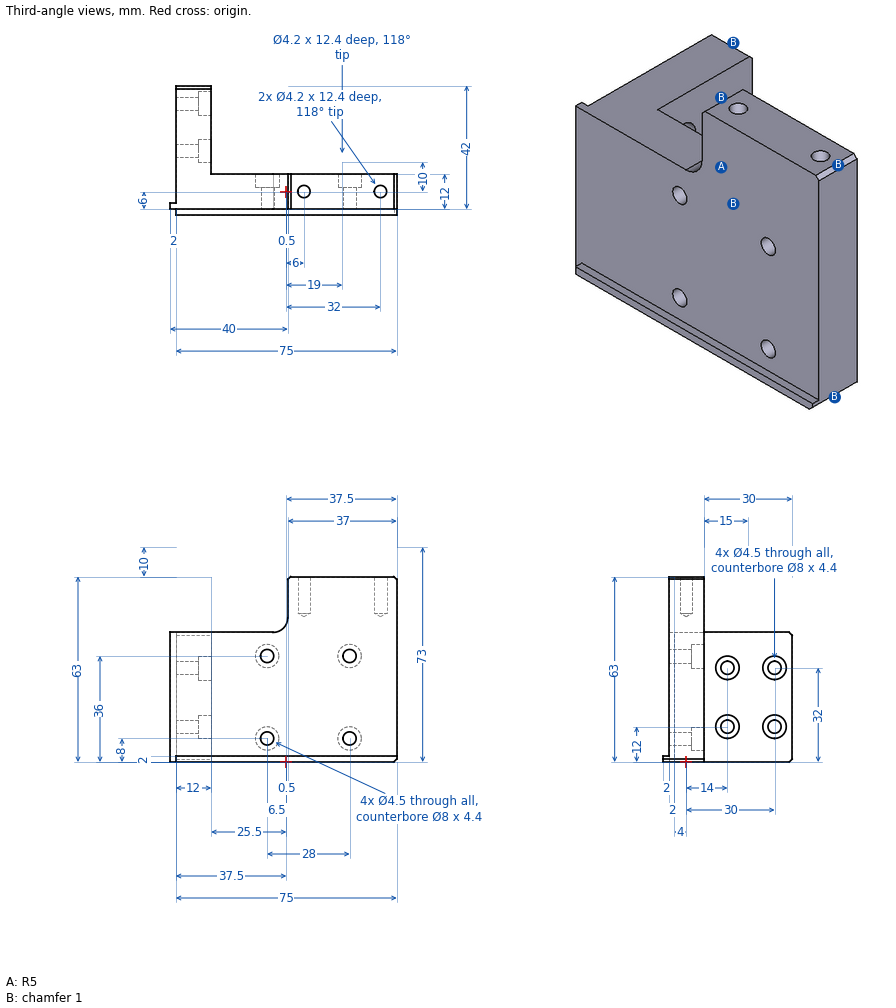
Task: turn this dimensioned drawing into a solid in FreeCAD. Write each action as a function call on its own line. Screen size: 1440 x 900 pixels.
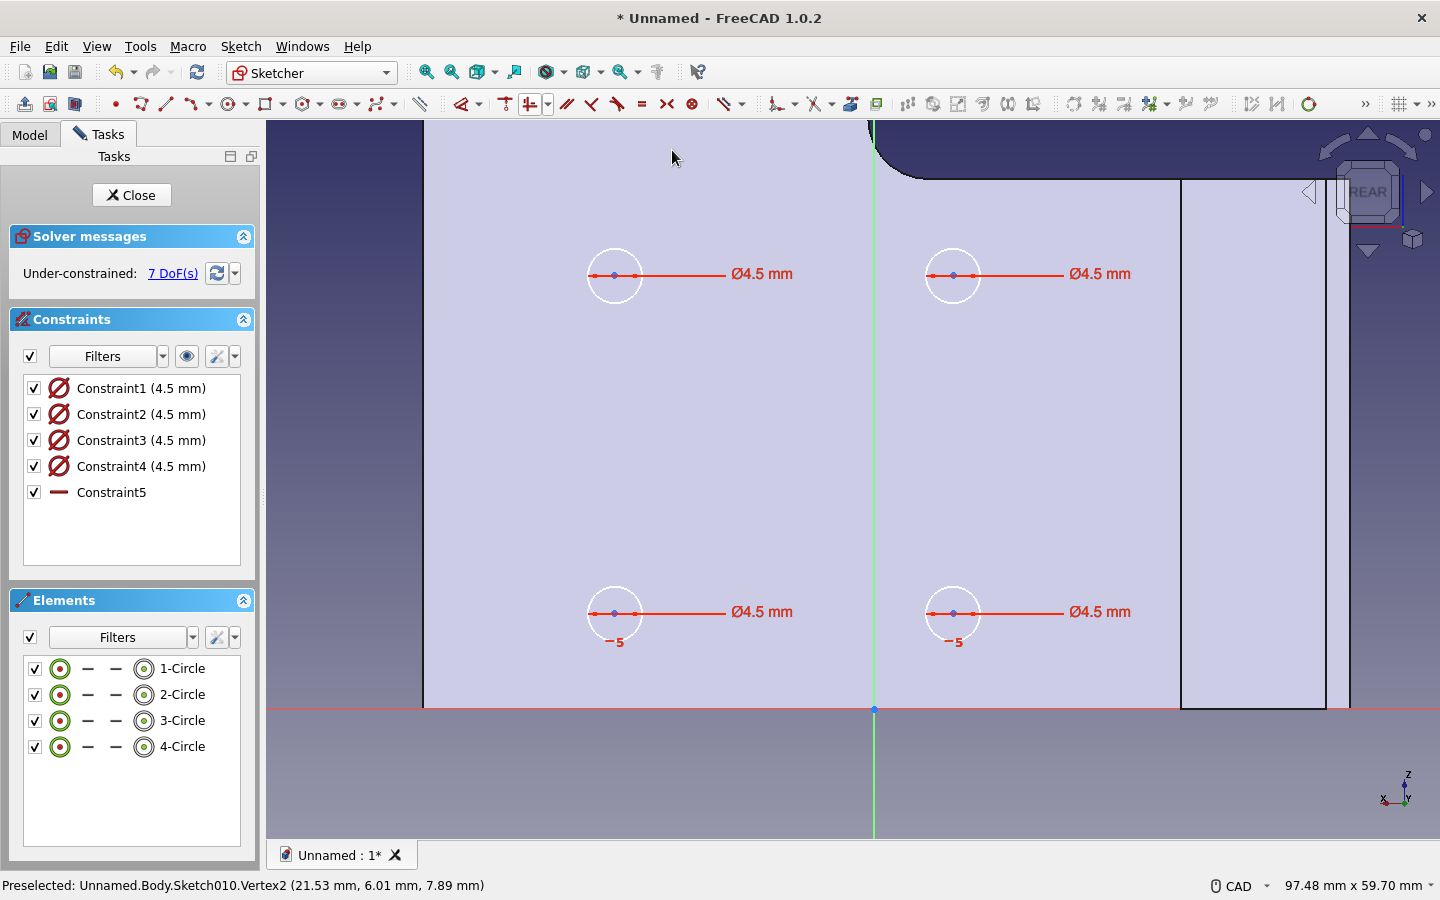
click(953, 614)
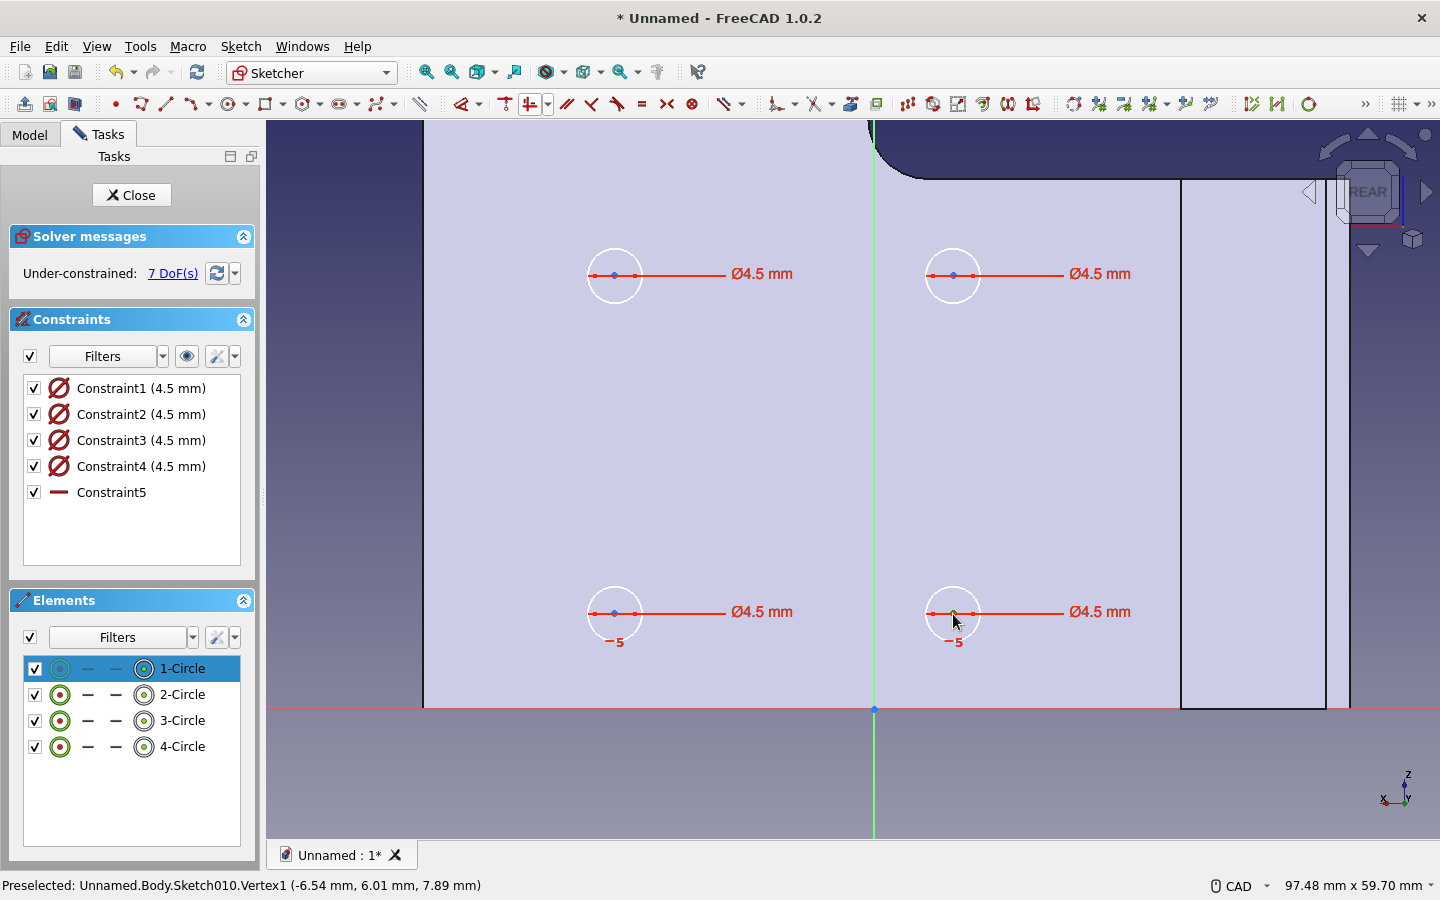
click(953, 276)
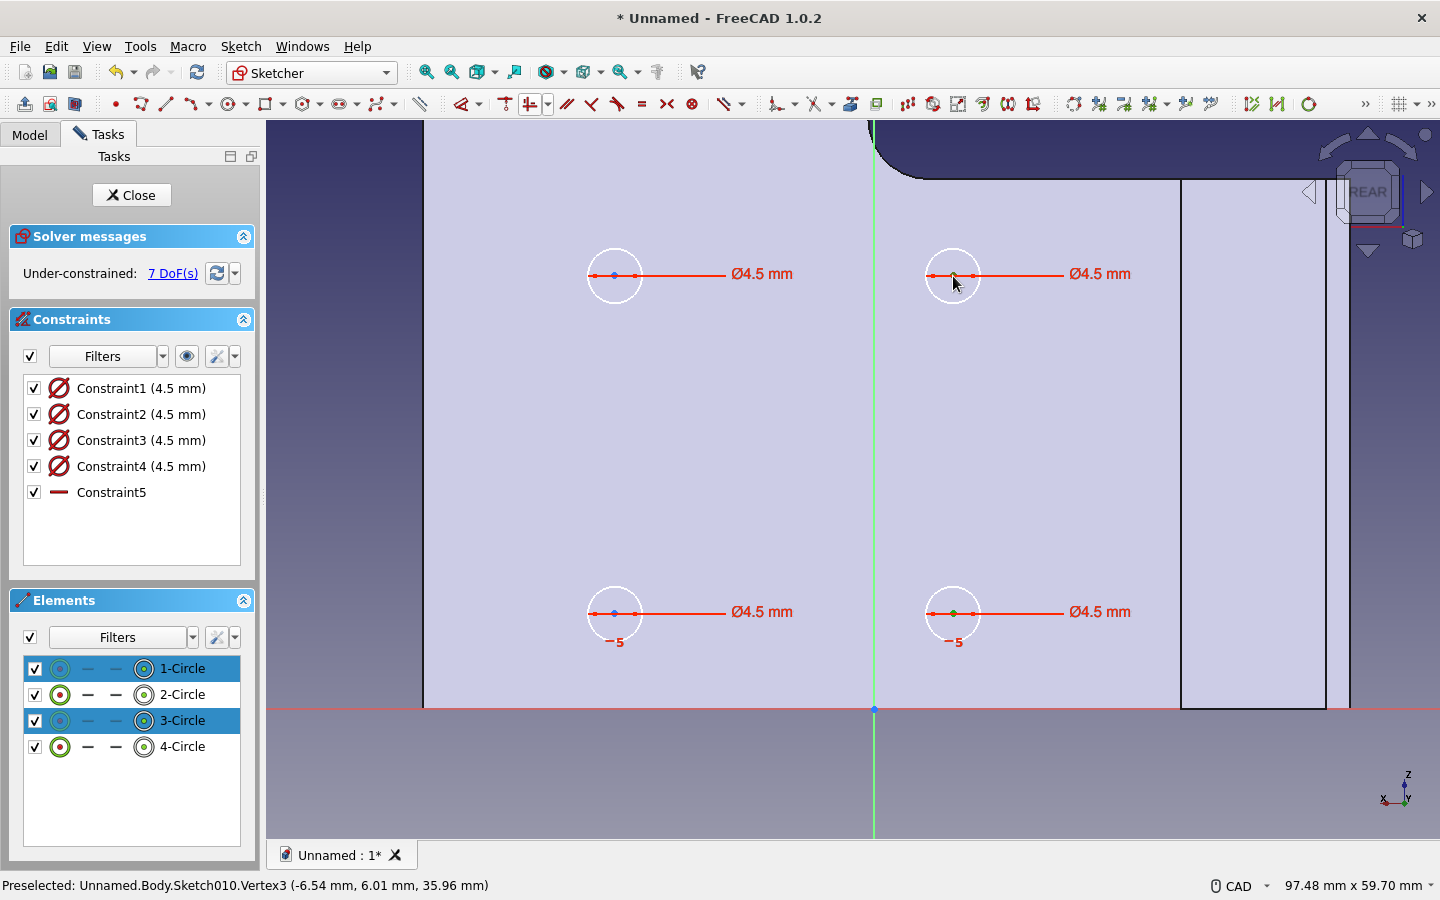
click(548, 104)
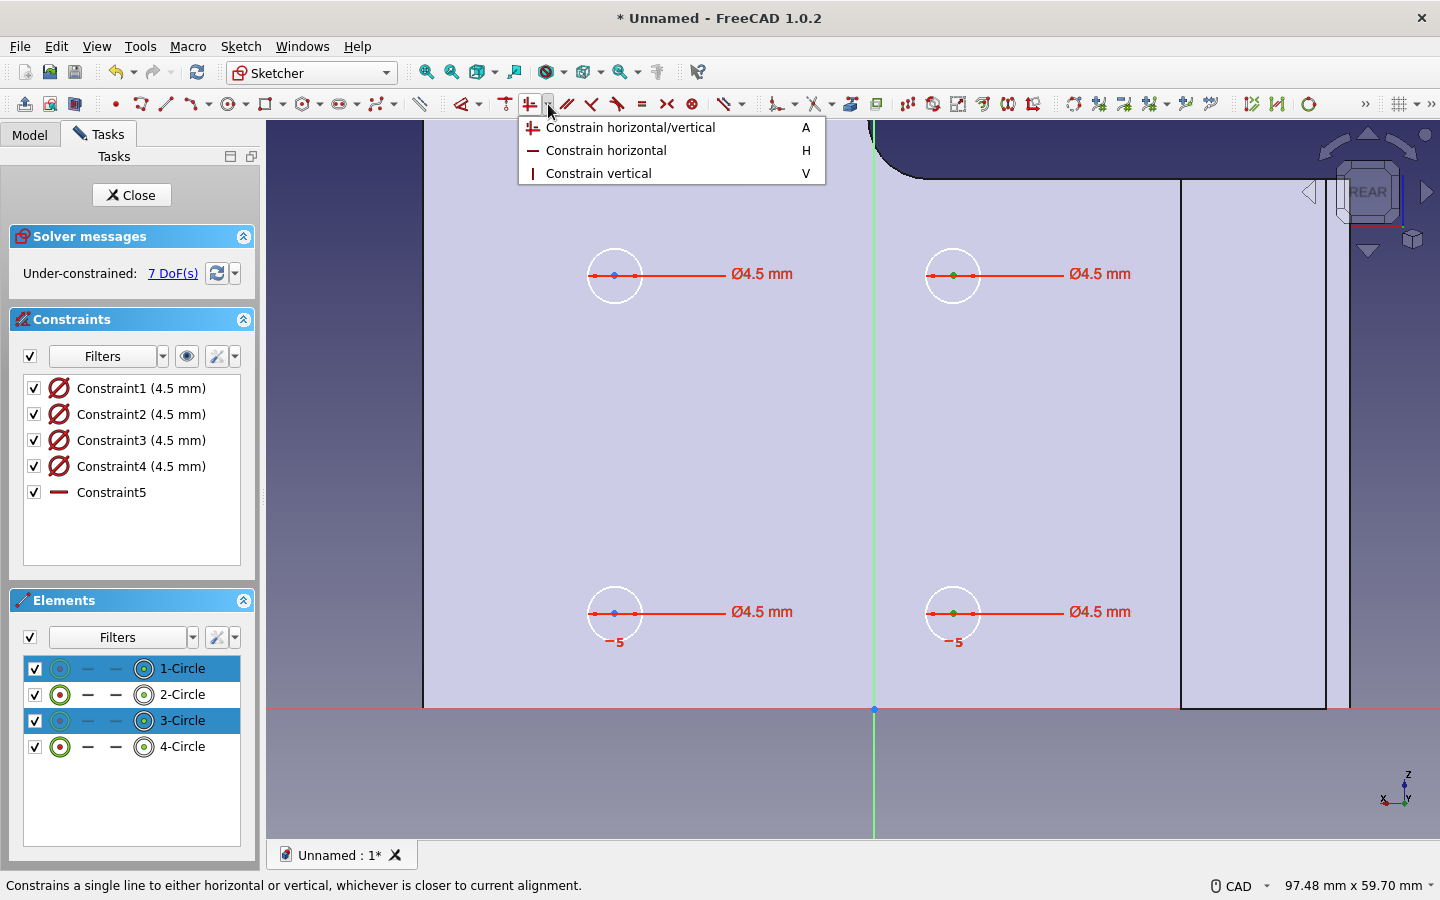
click(672, 174)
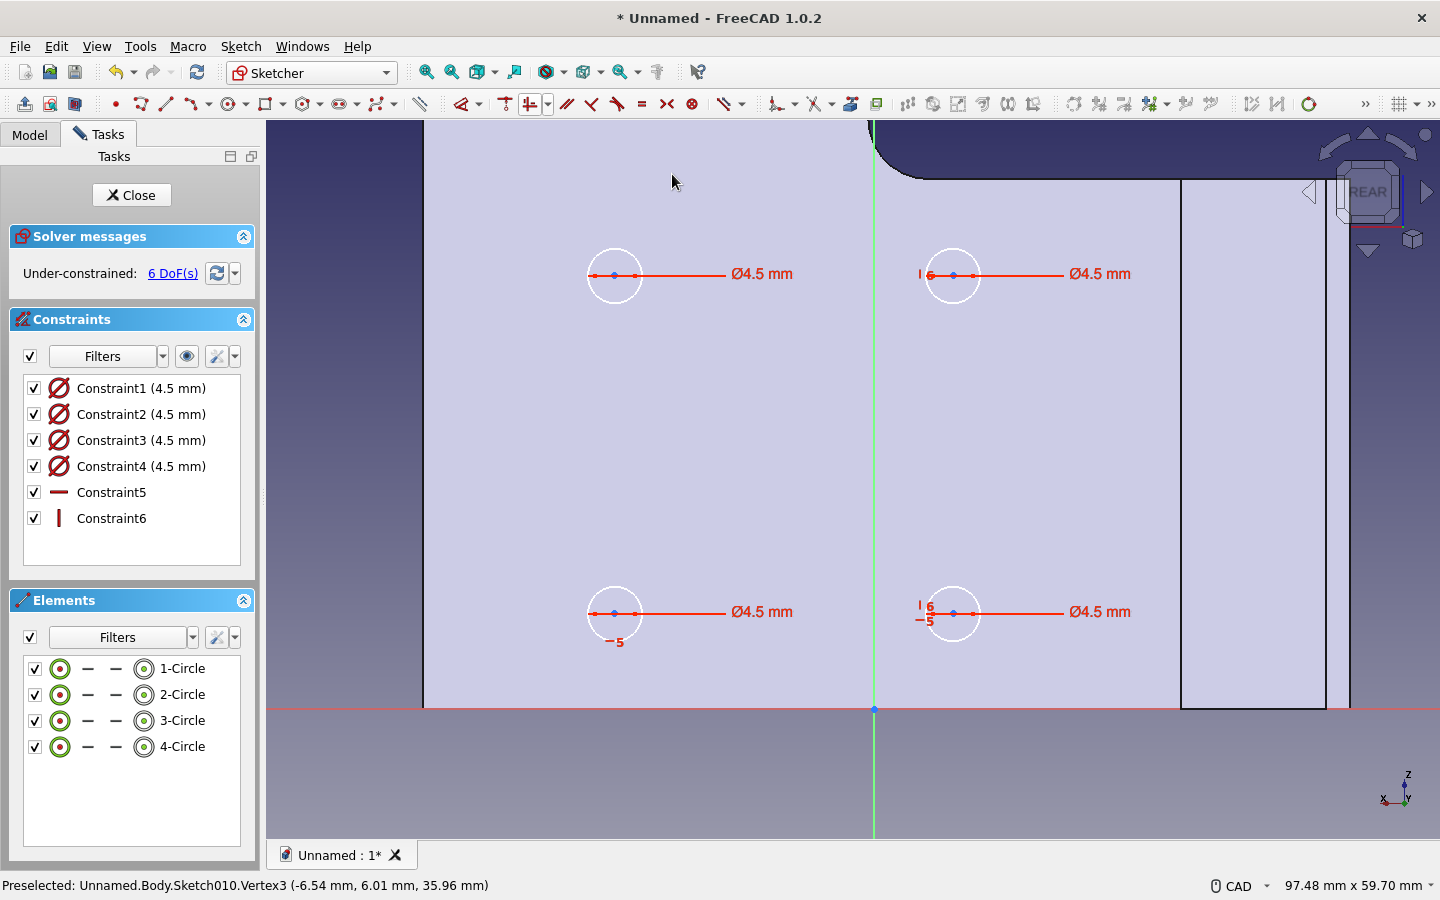
click(615, 614)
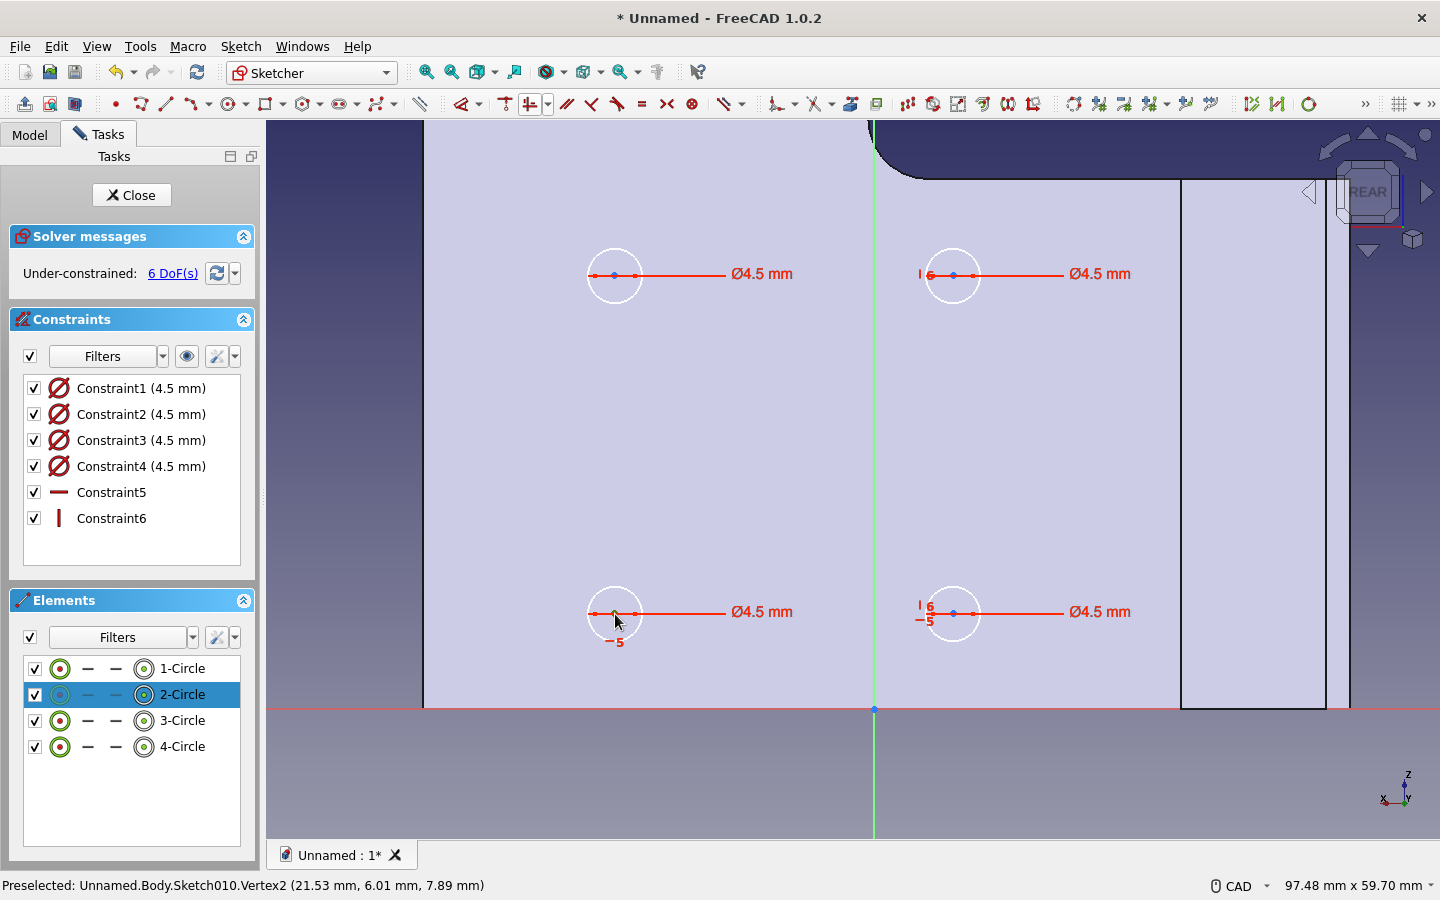
click(615, 276)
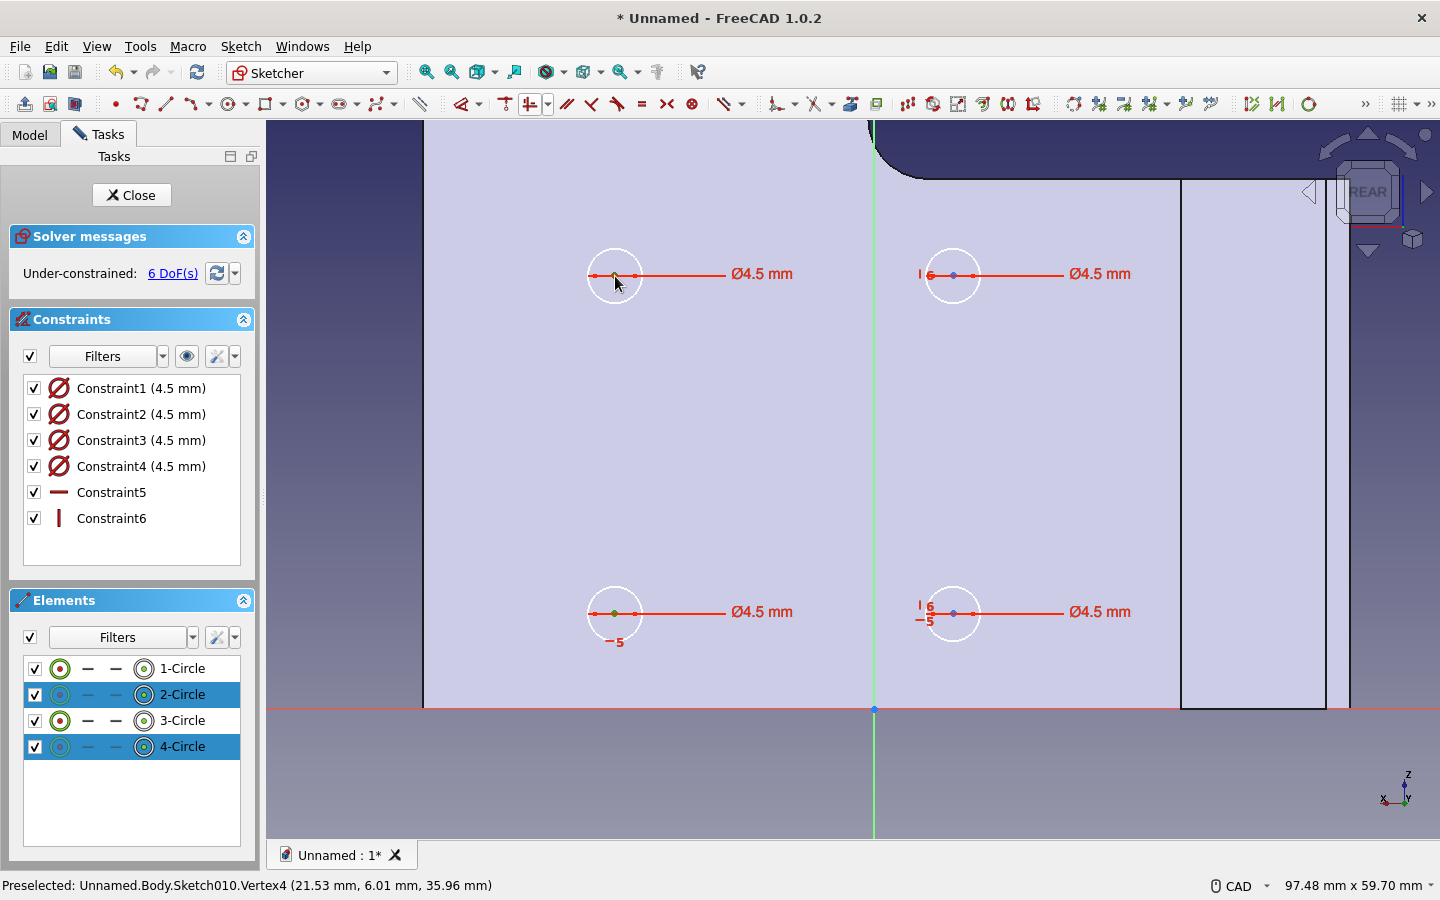
key(v)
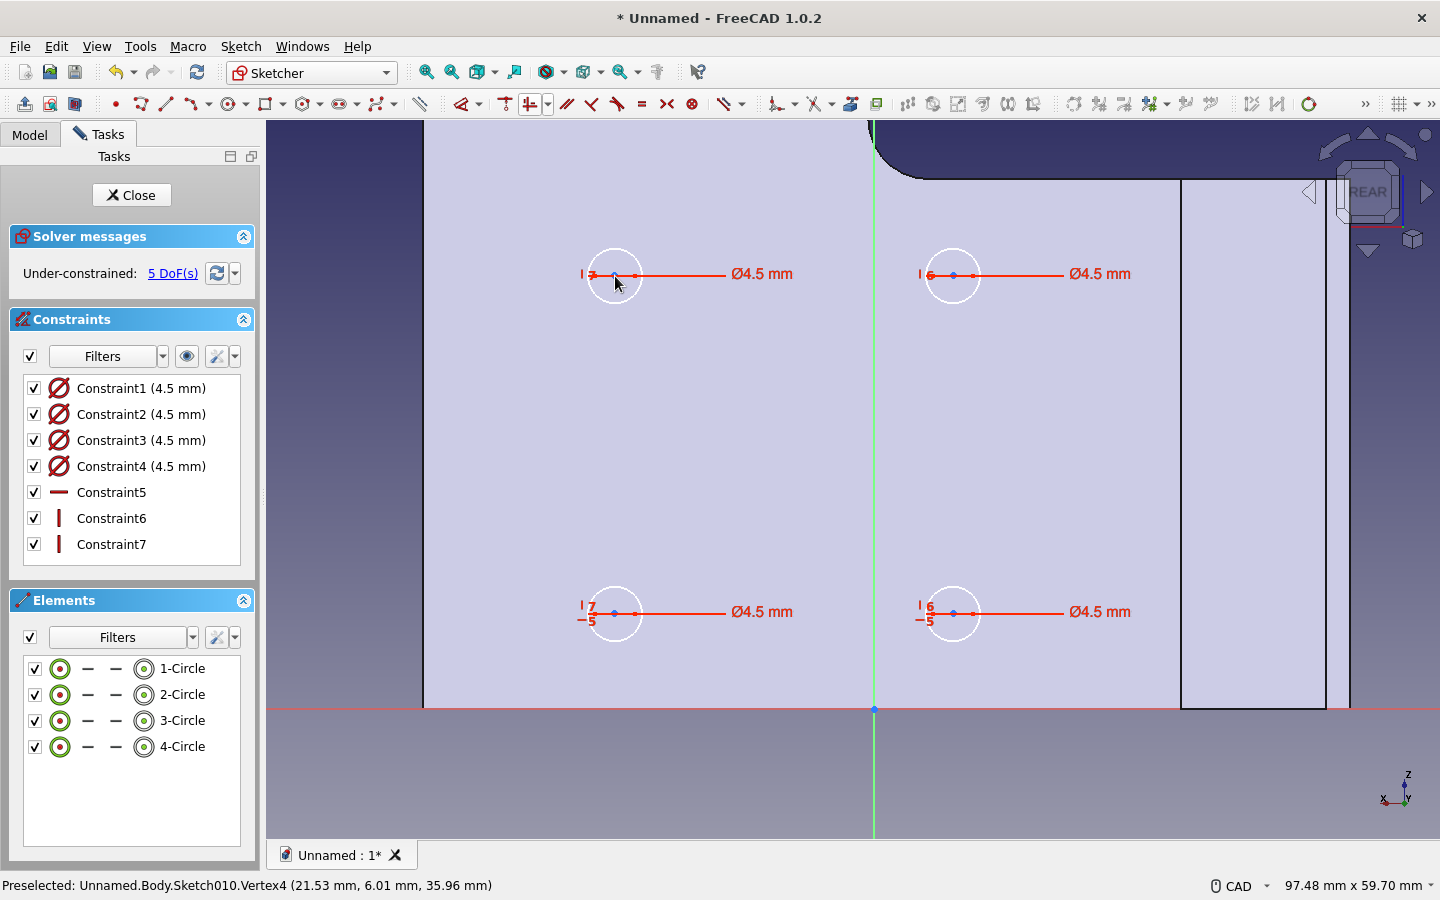
click(953, 276)